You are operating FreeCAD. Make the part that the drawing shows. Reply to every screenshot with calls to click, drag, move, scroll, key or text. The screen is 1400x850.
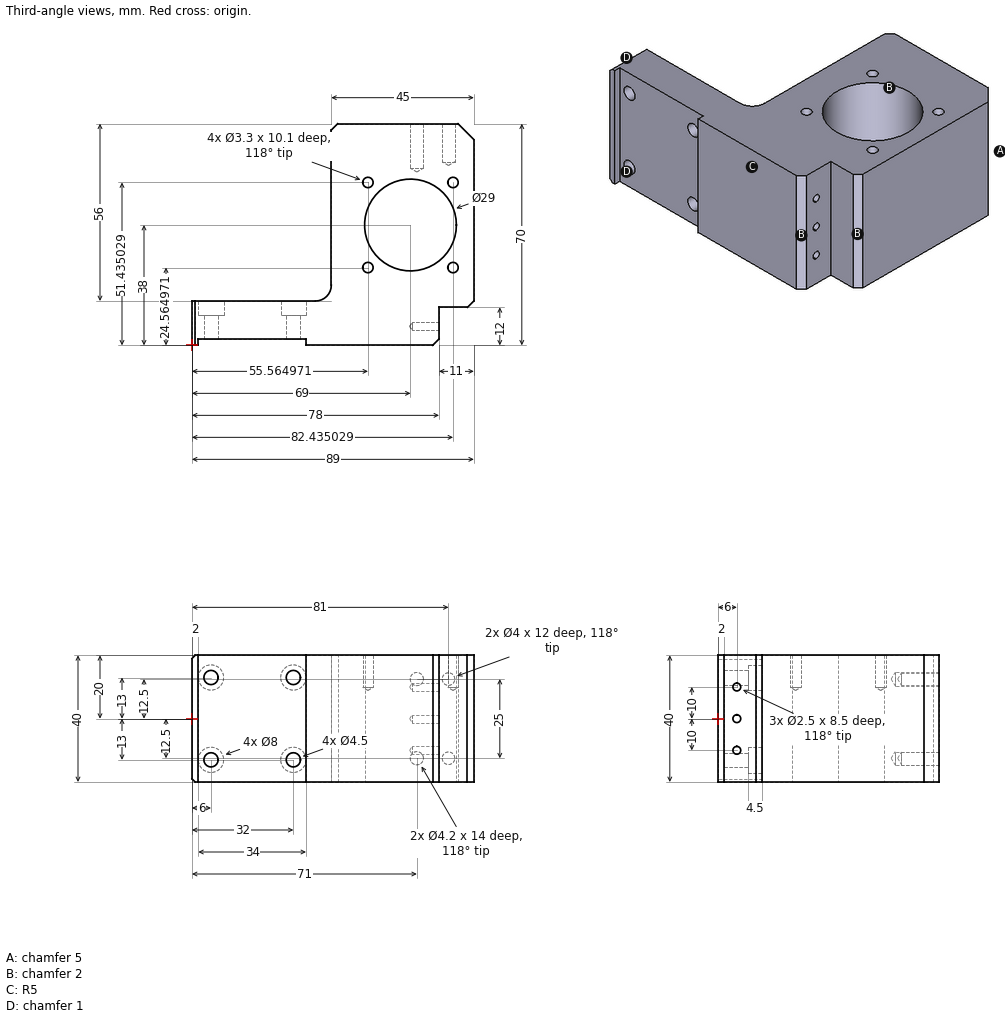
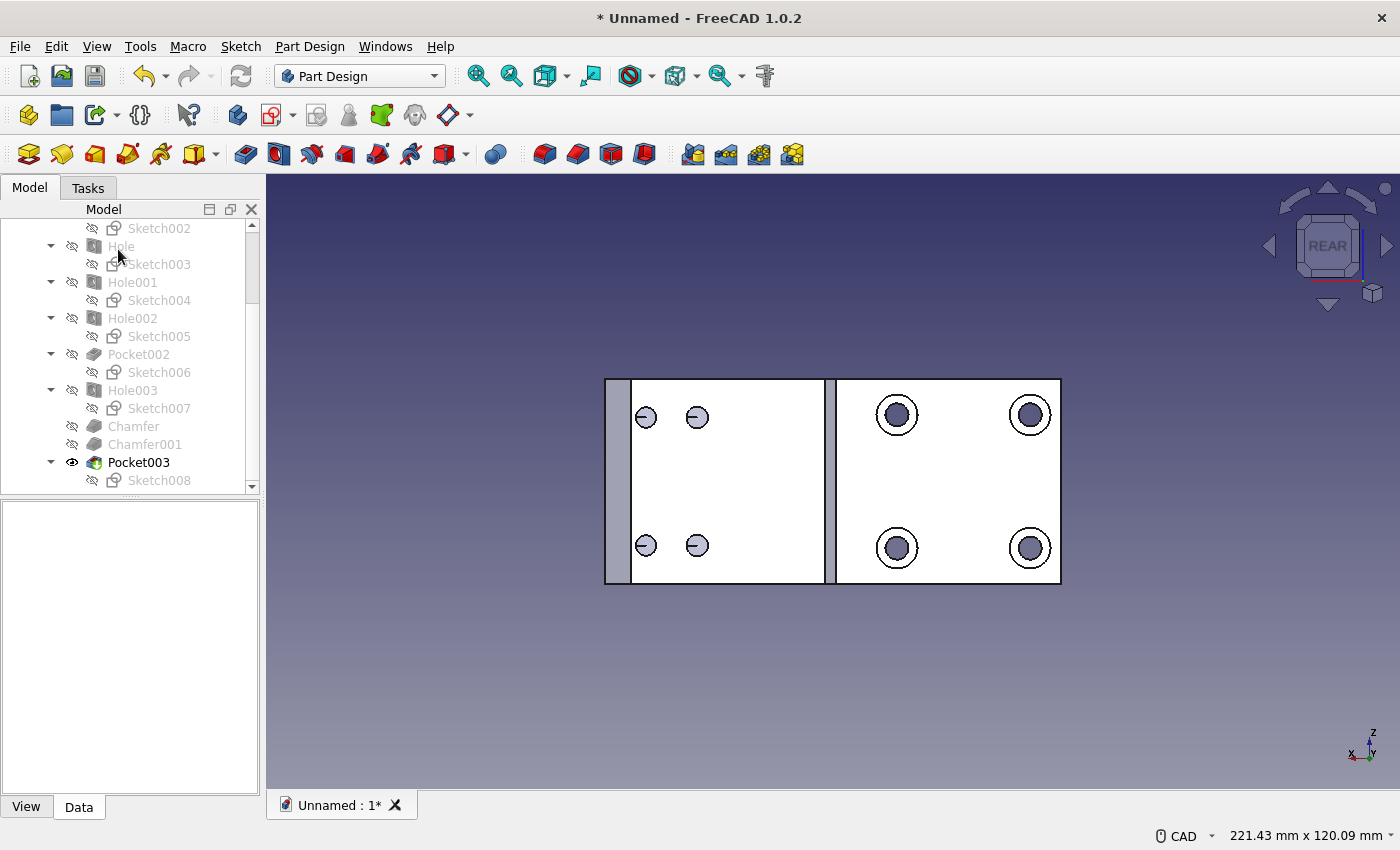
click(479, 76)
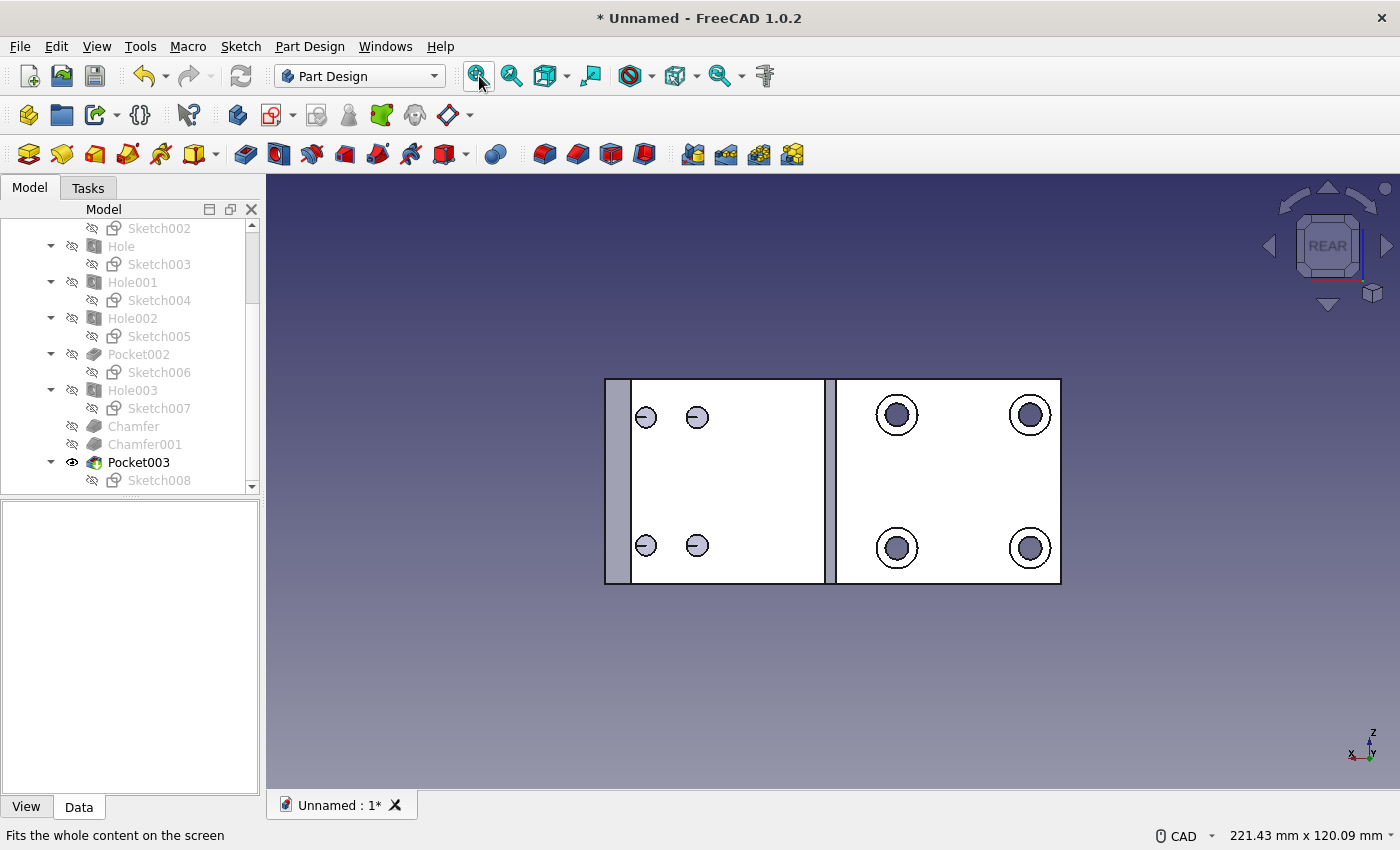
key(0)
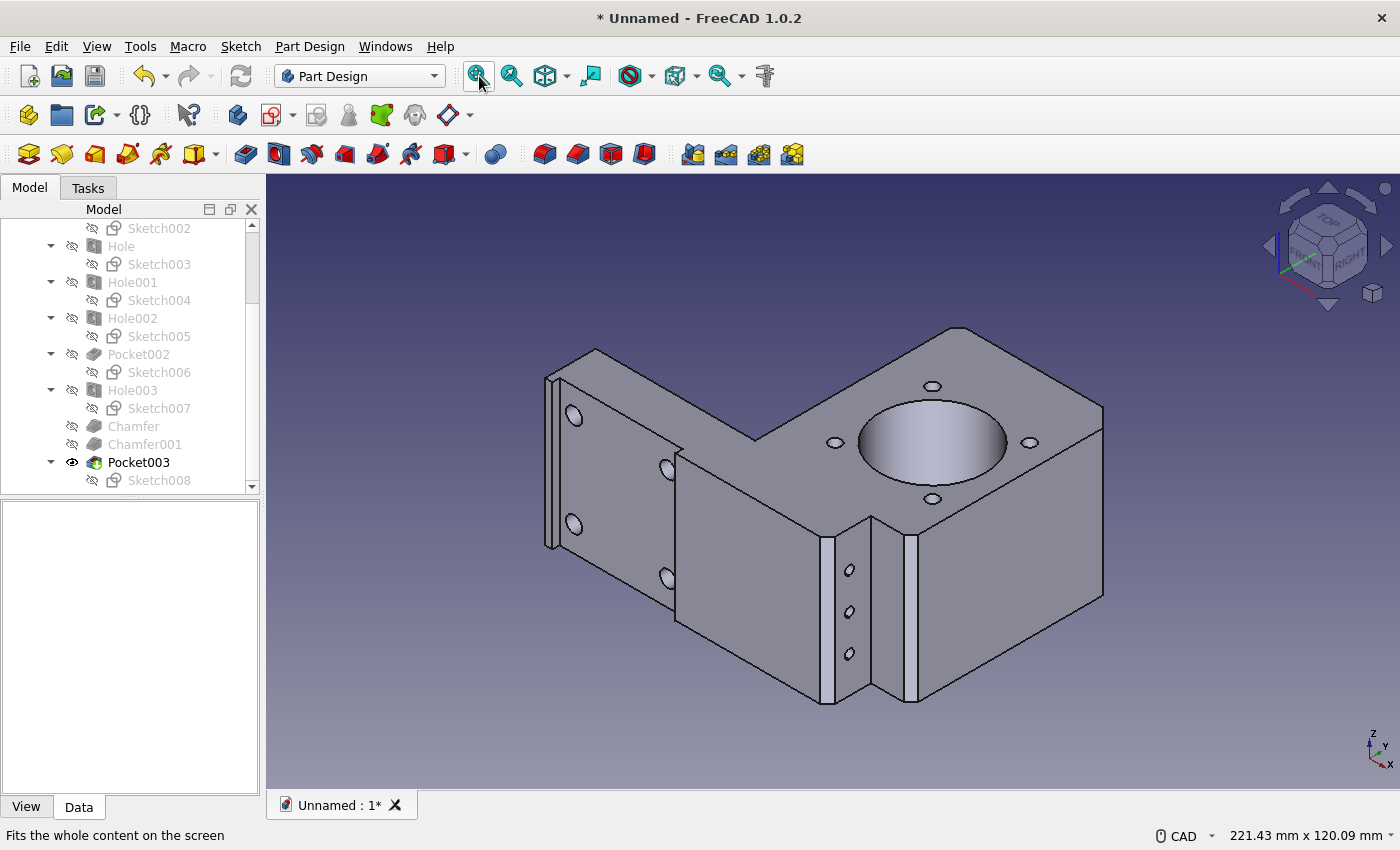
key(2)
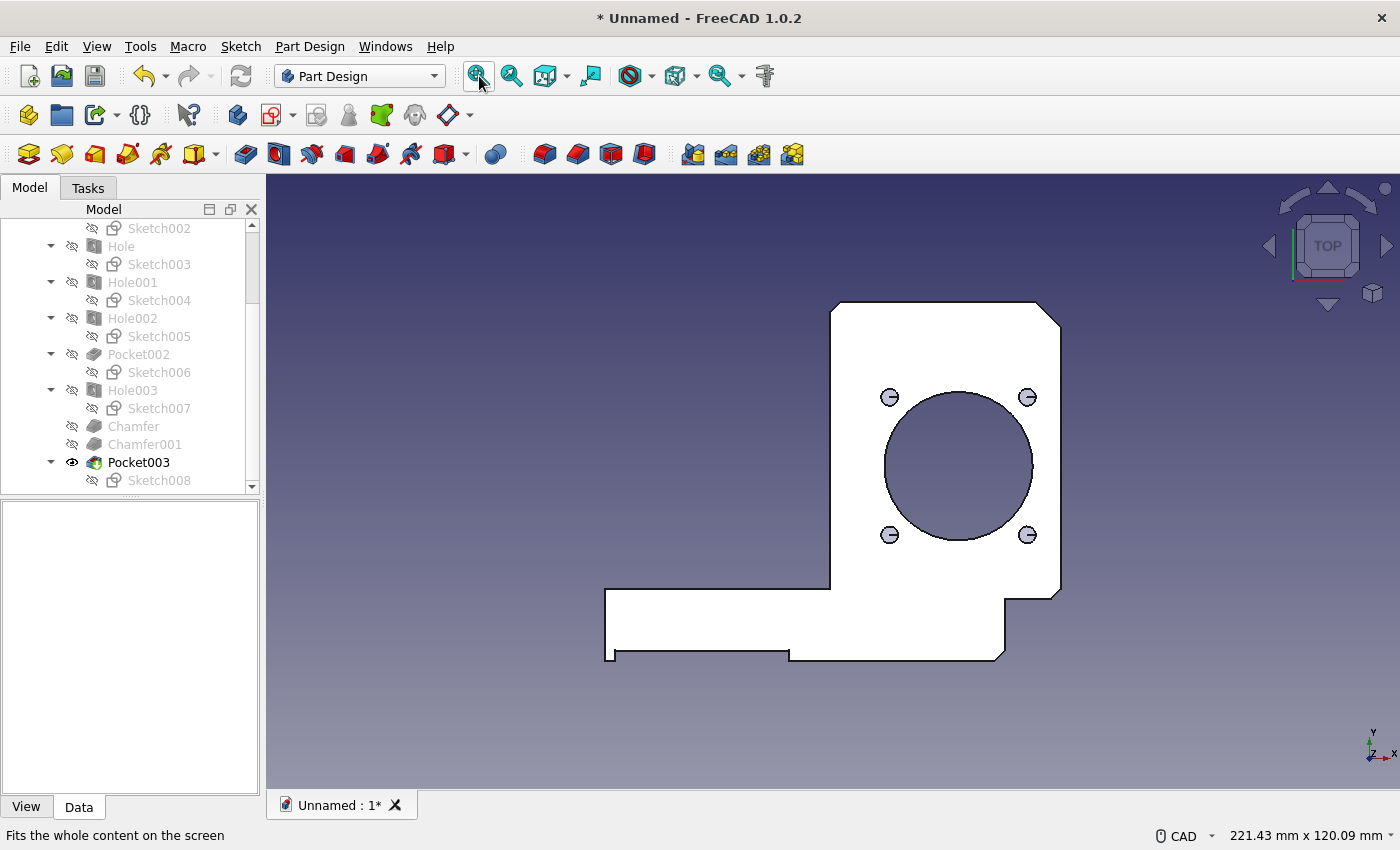
key(1)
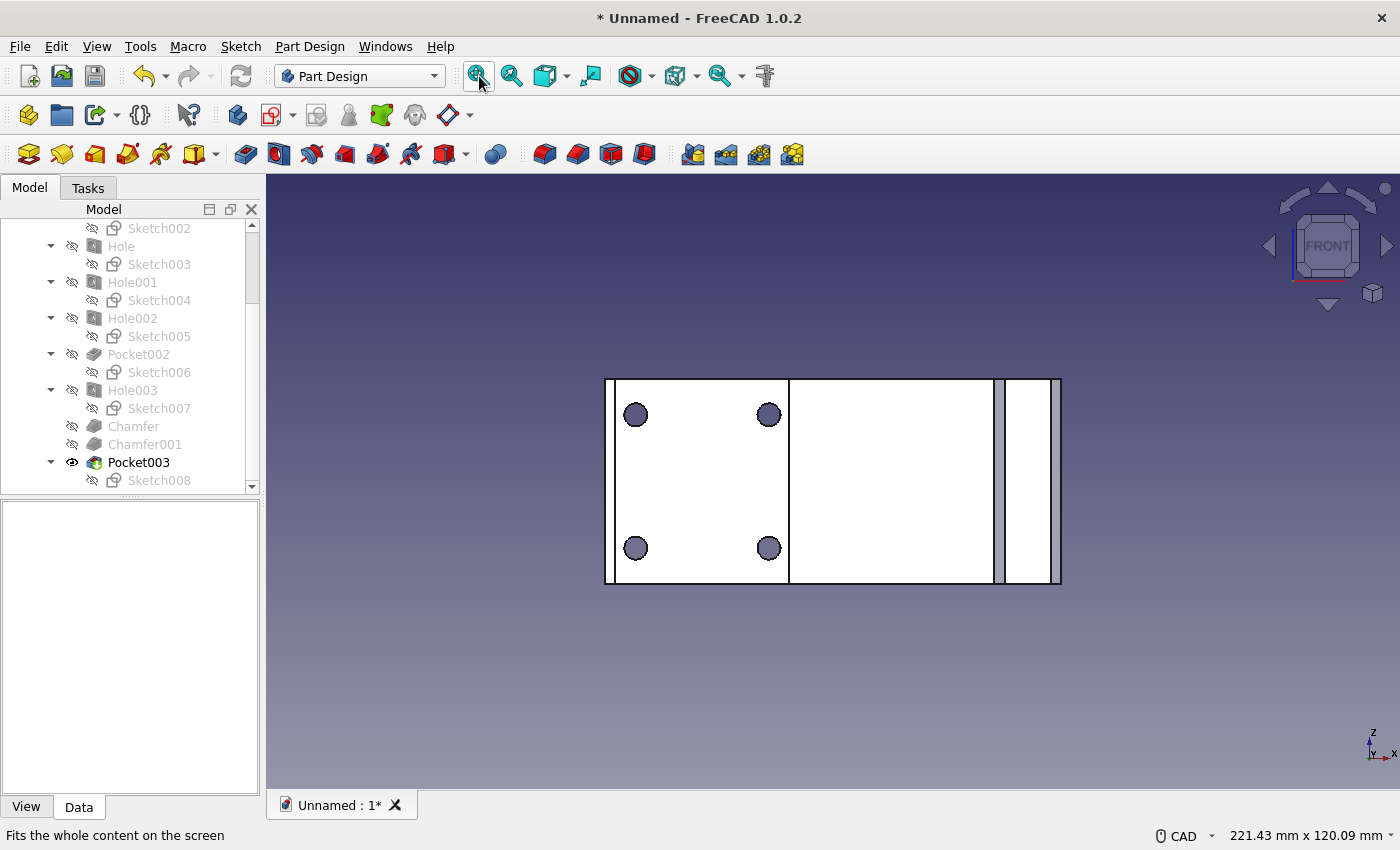
click(479, 76)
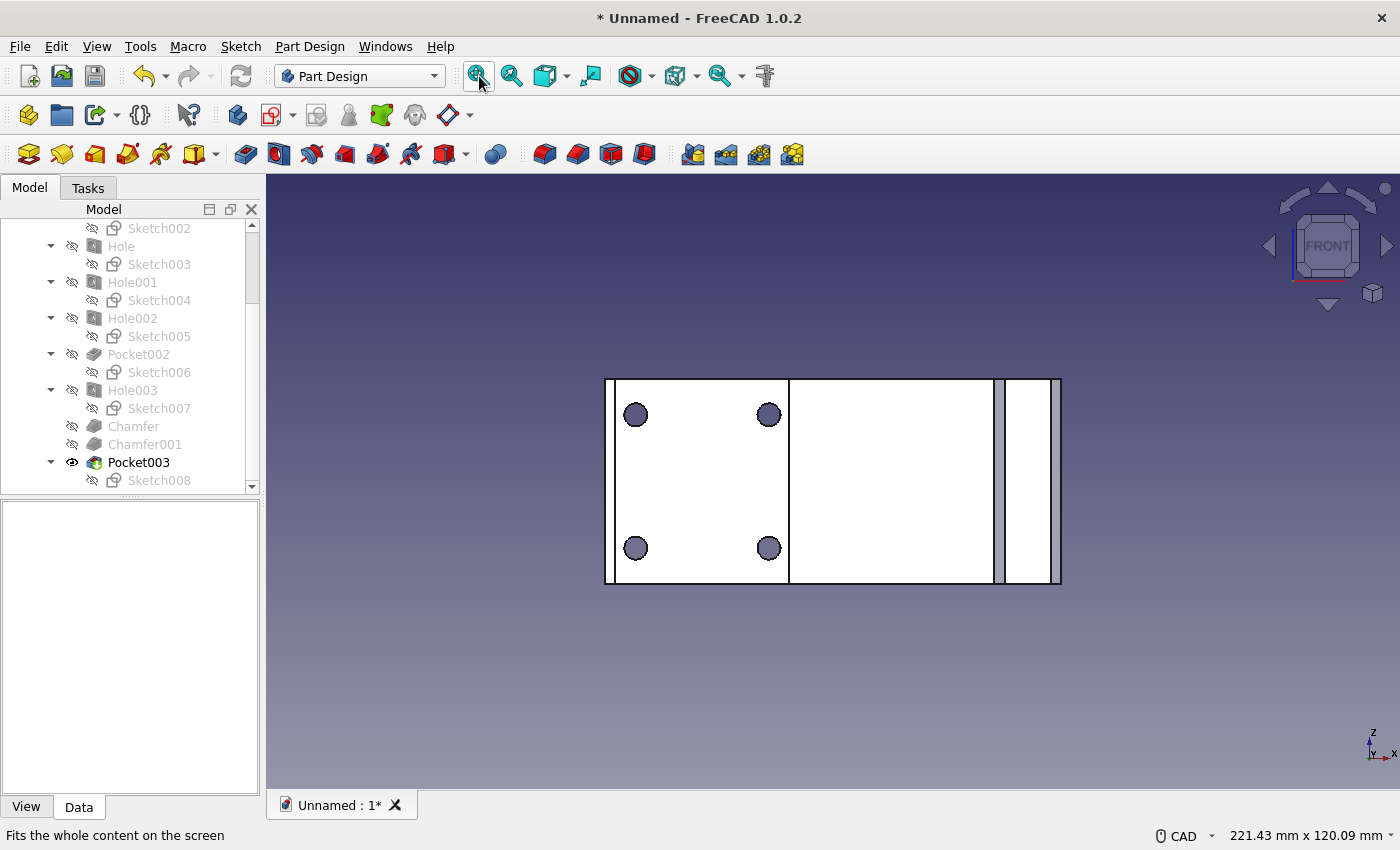
key(3)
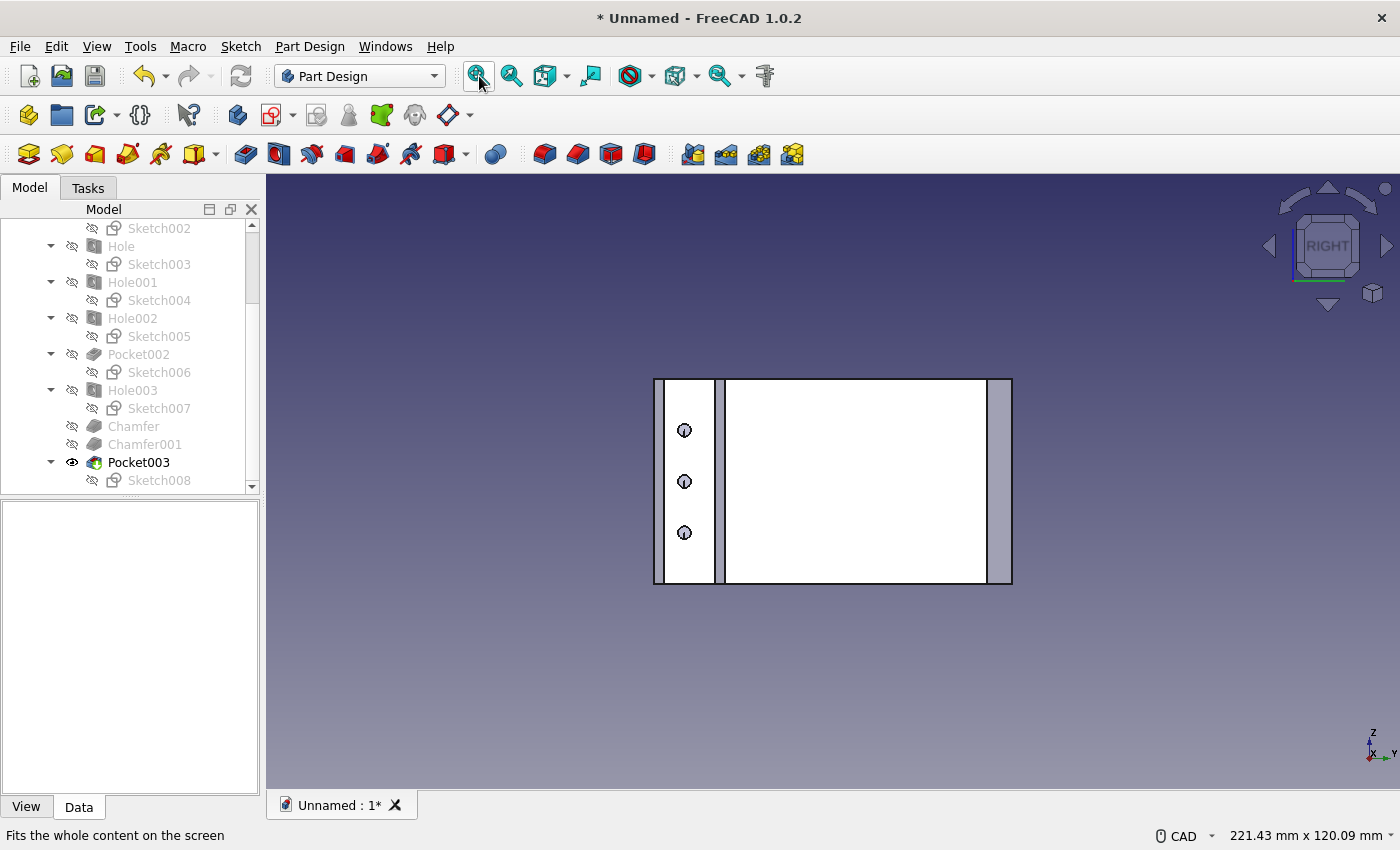
click(479, 76)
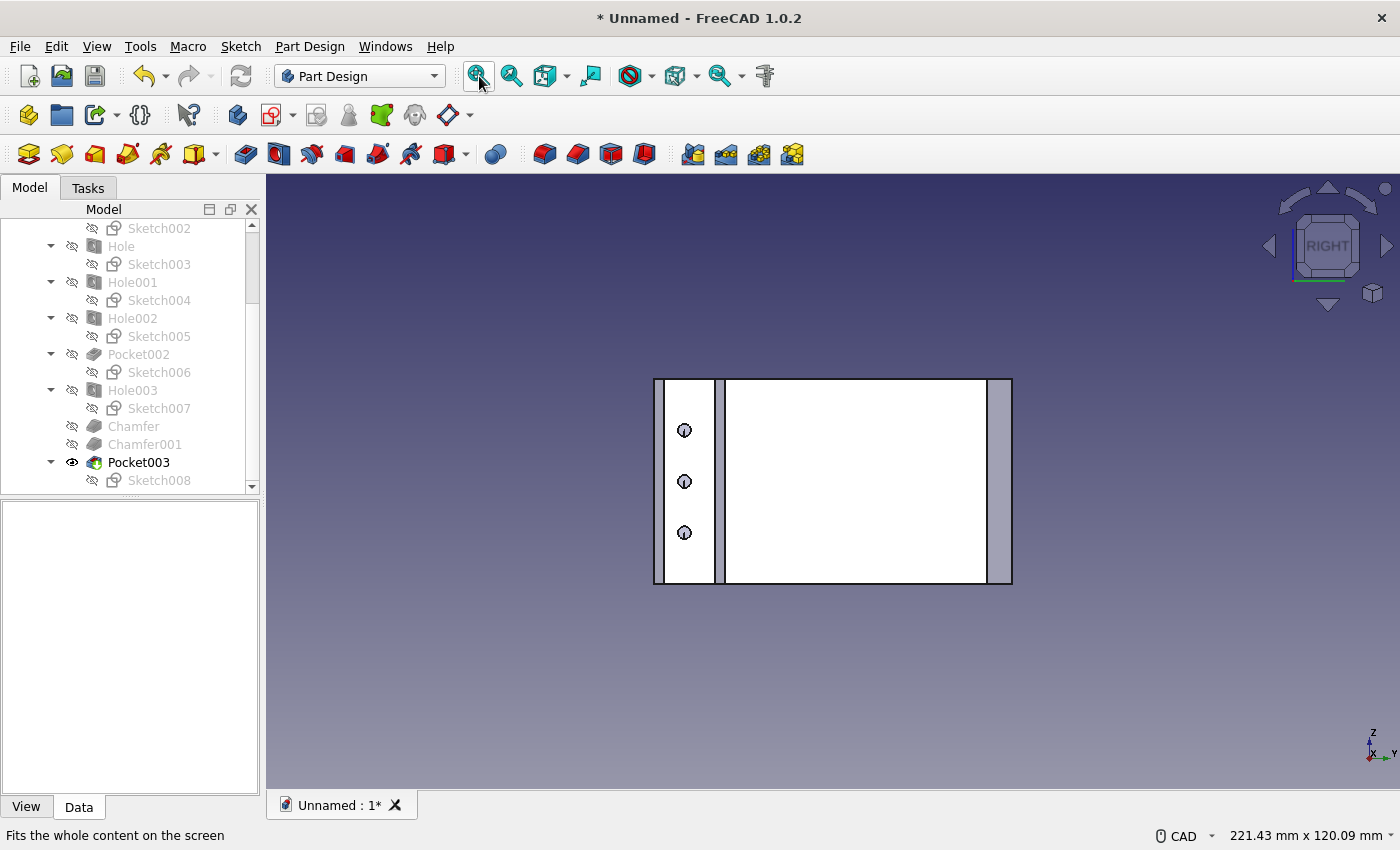
key(5)